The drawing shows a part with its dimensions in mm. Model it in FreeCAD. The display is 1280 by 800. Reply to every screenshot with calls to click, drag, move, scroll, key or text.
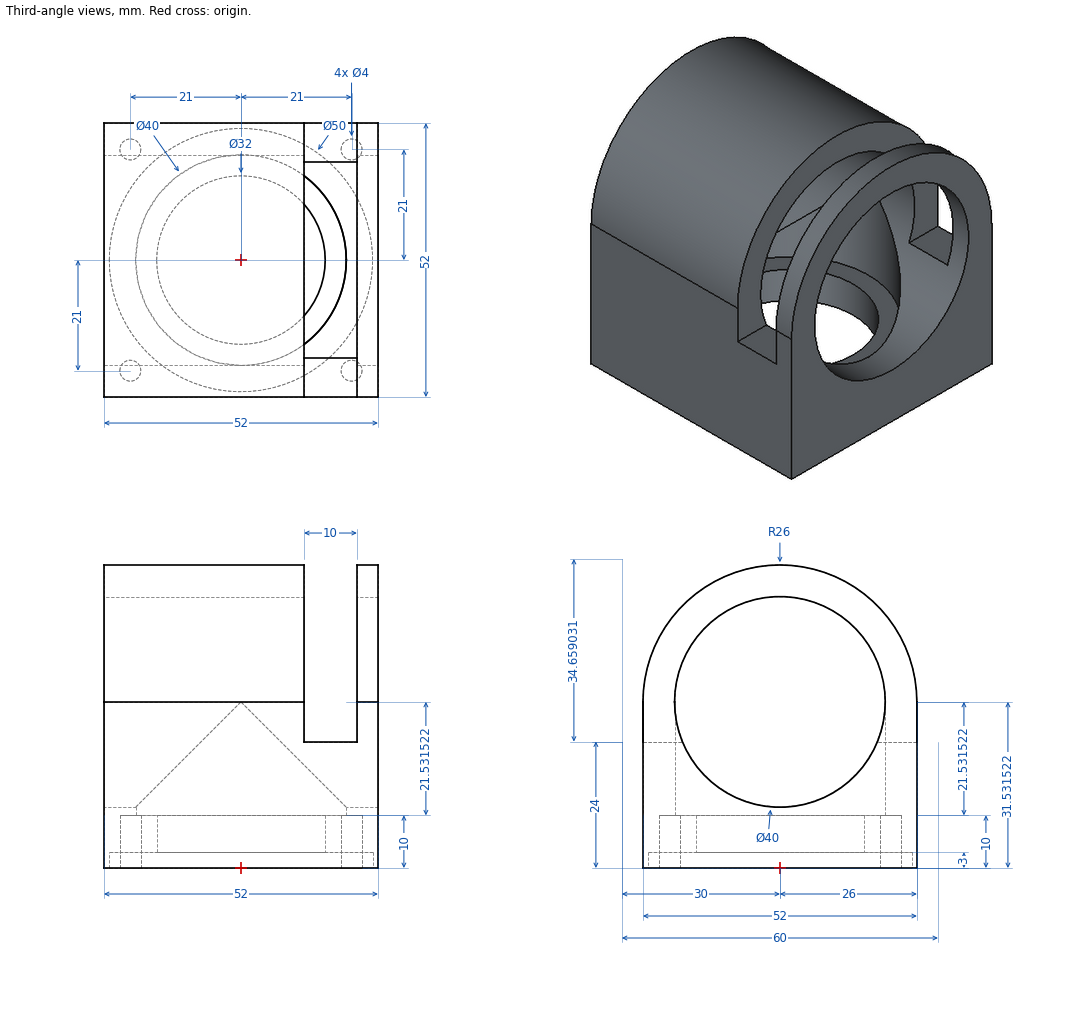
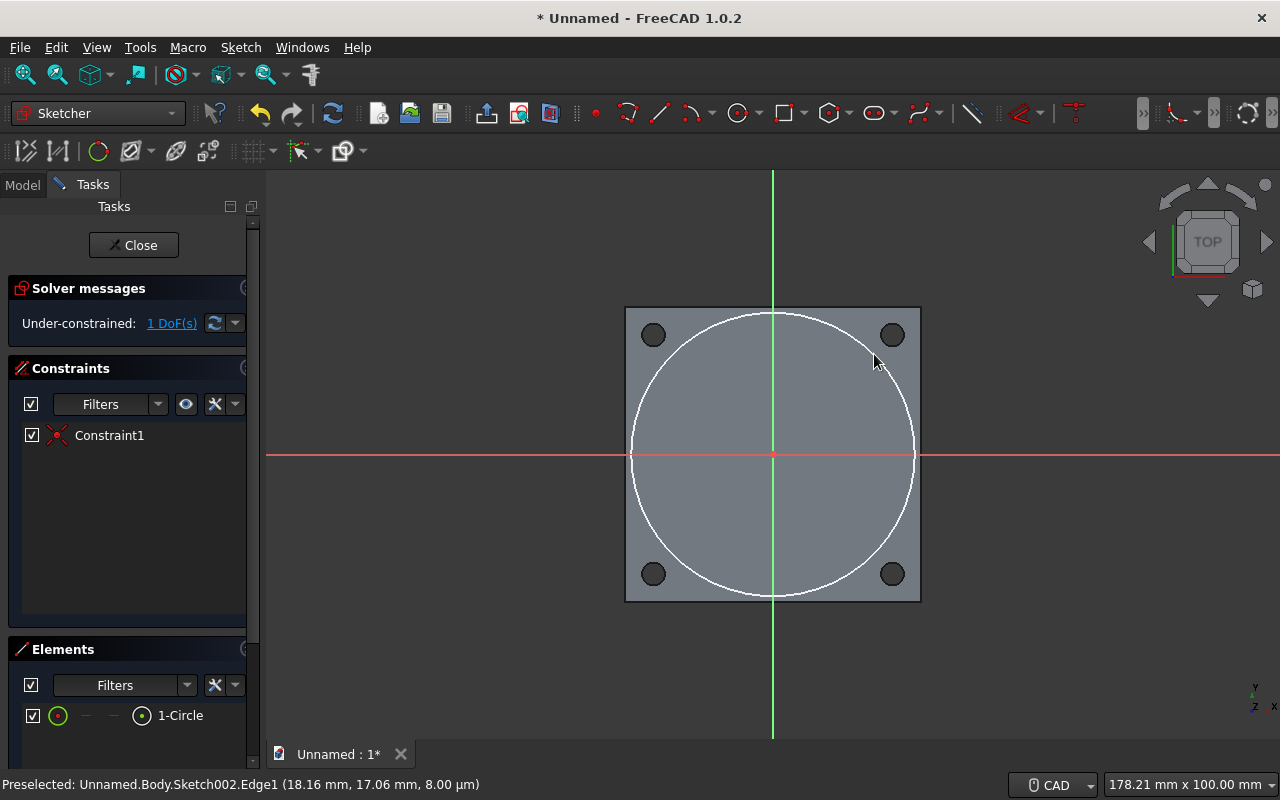
click(1020, 114)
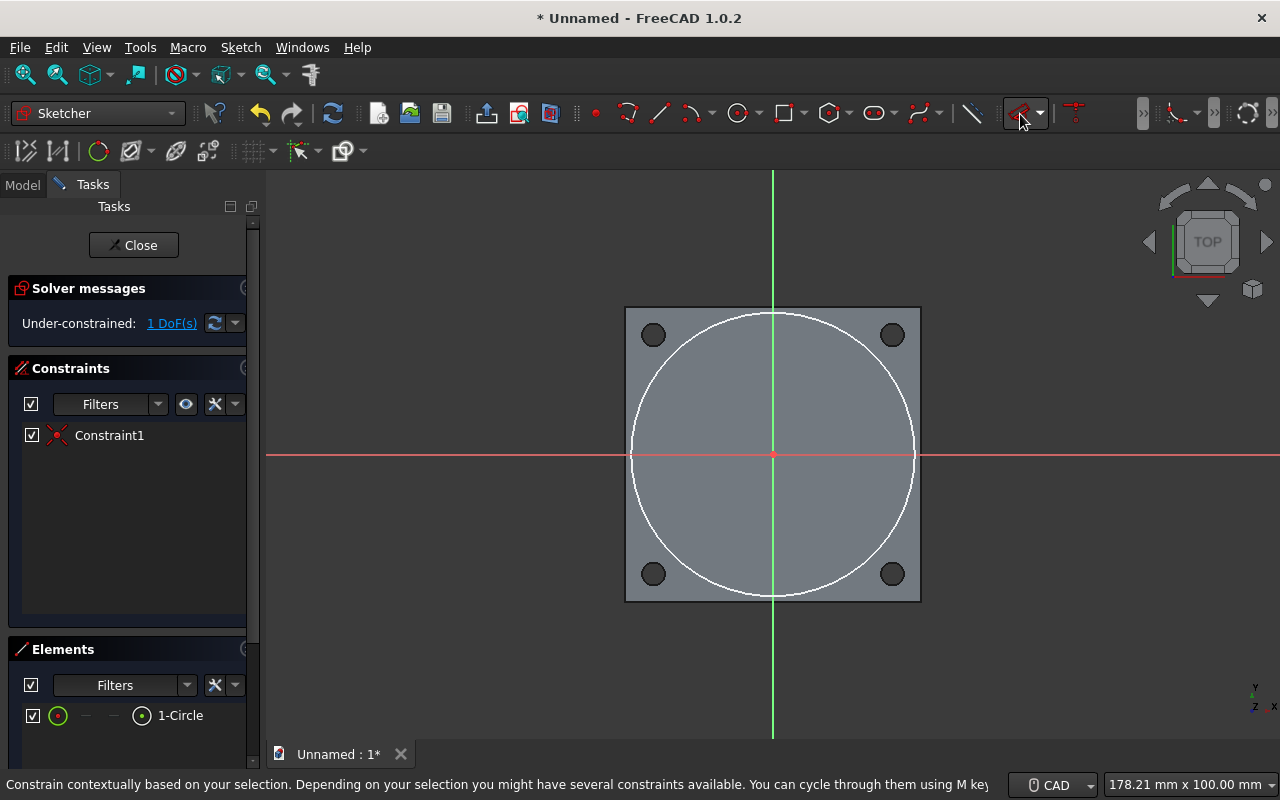
click(873, 354)
click(896, 331)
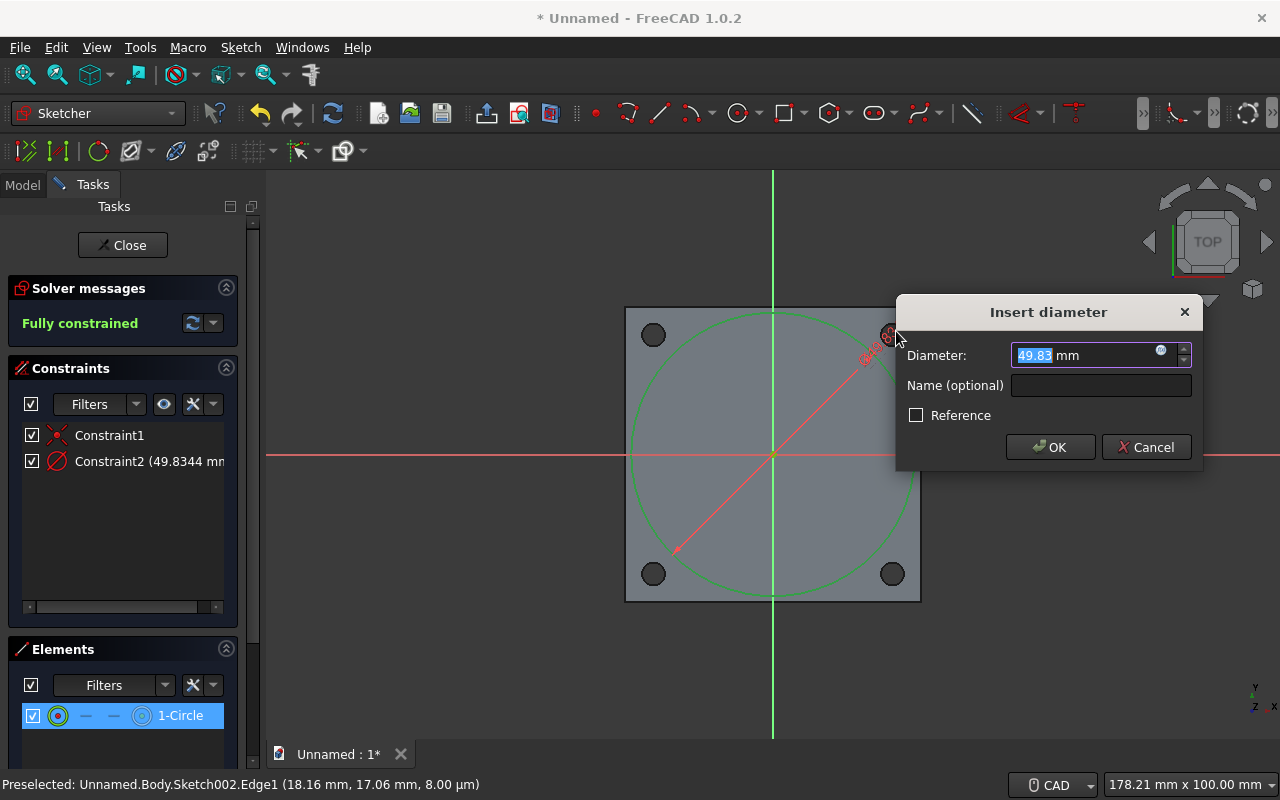
text(50)
key(Return)
key(Escape)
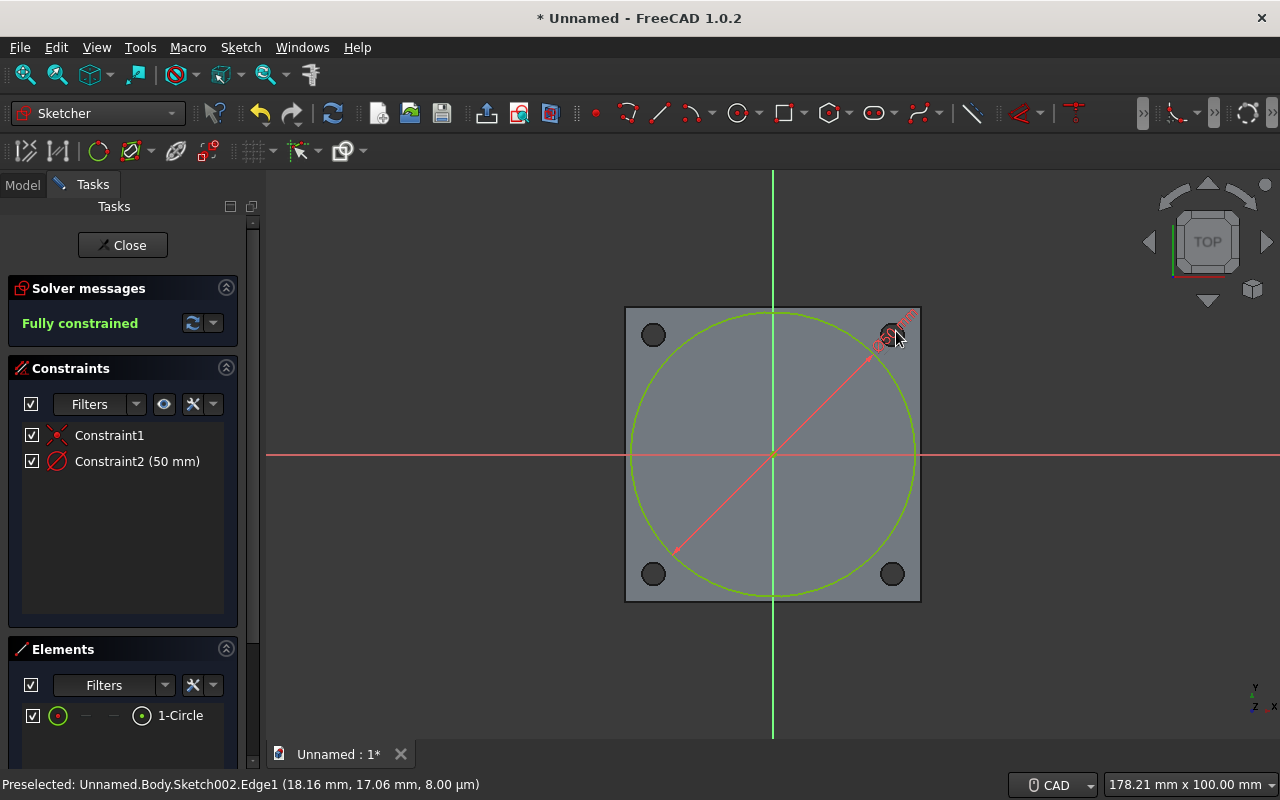
click(123, 245)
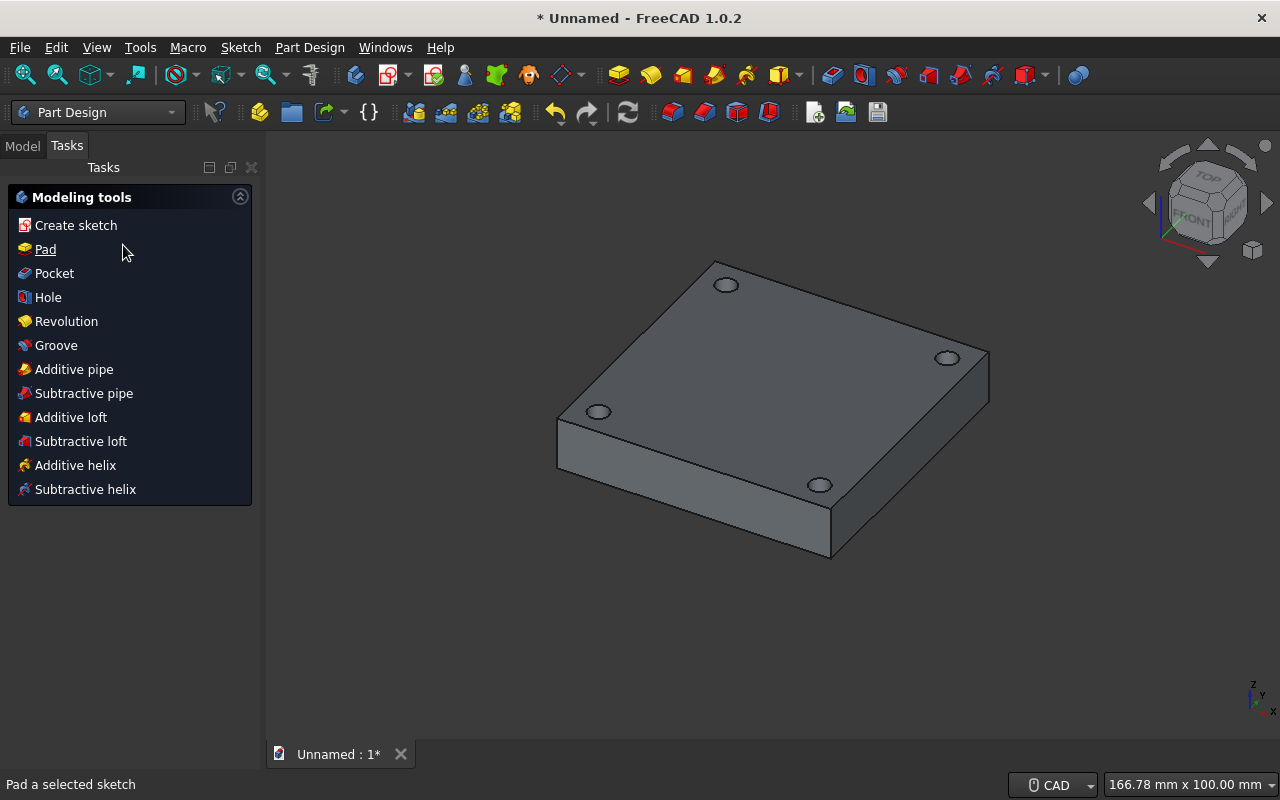
click(834, 76)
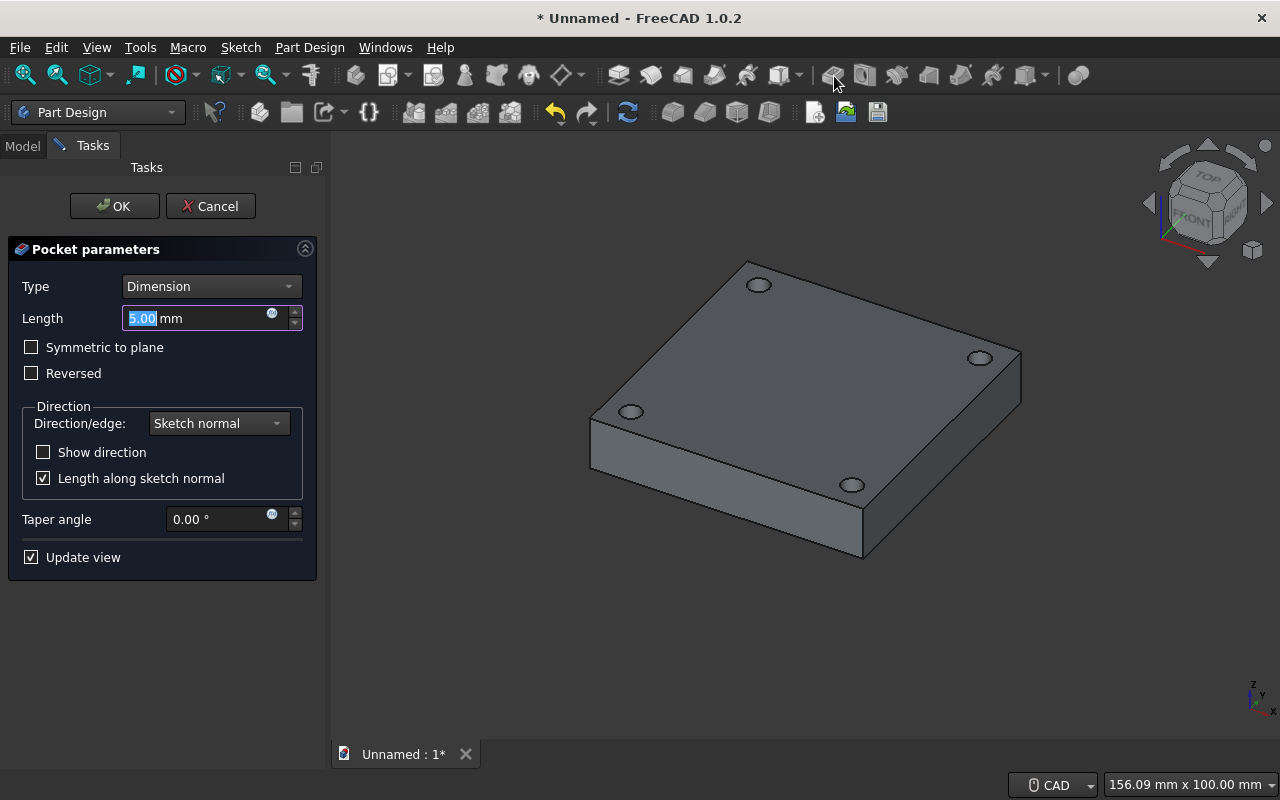
text(3)
key(Tab)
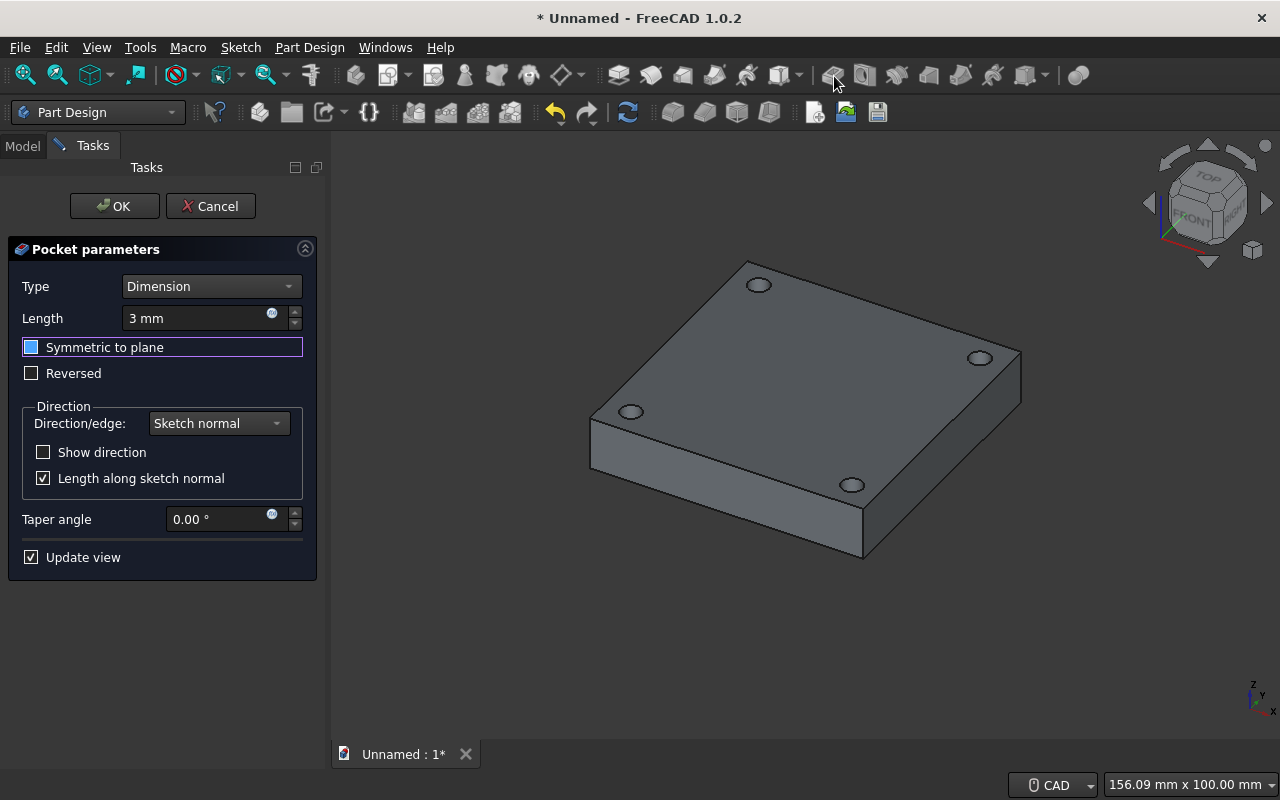
click(30, 373)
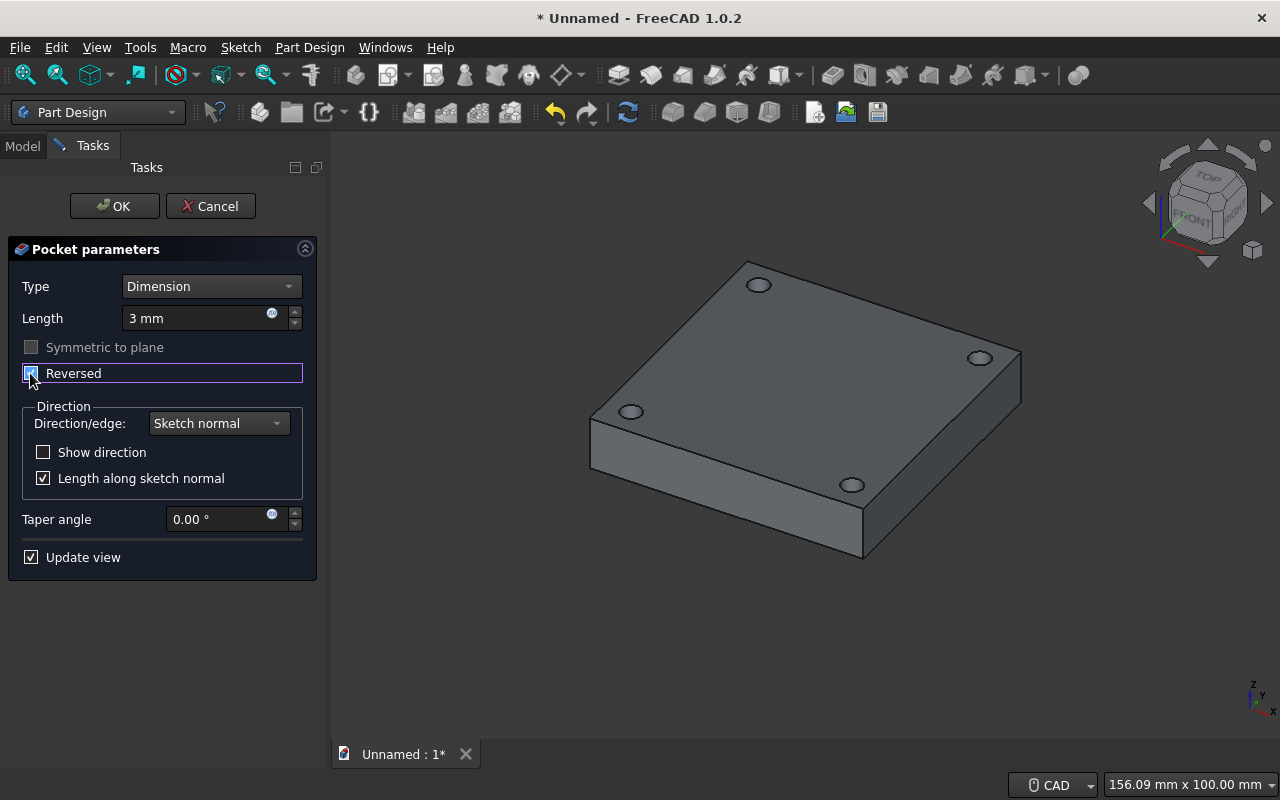
click(115, 206)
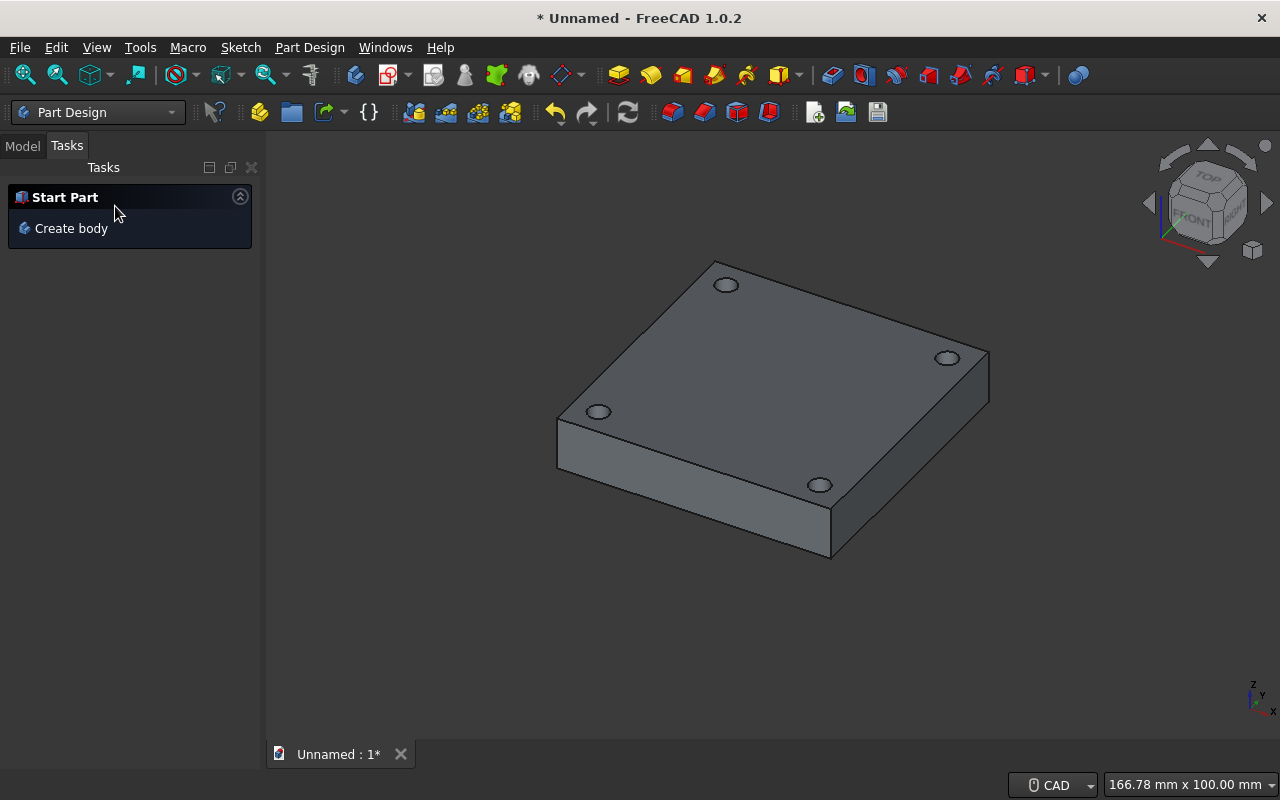
key(5)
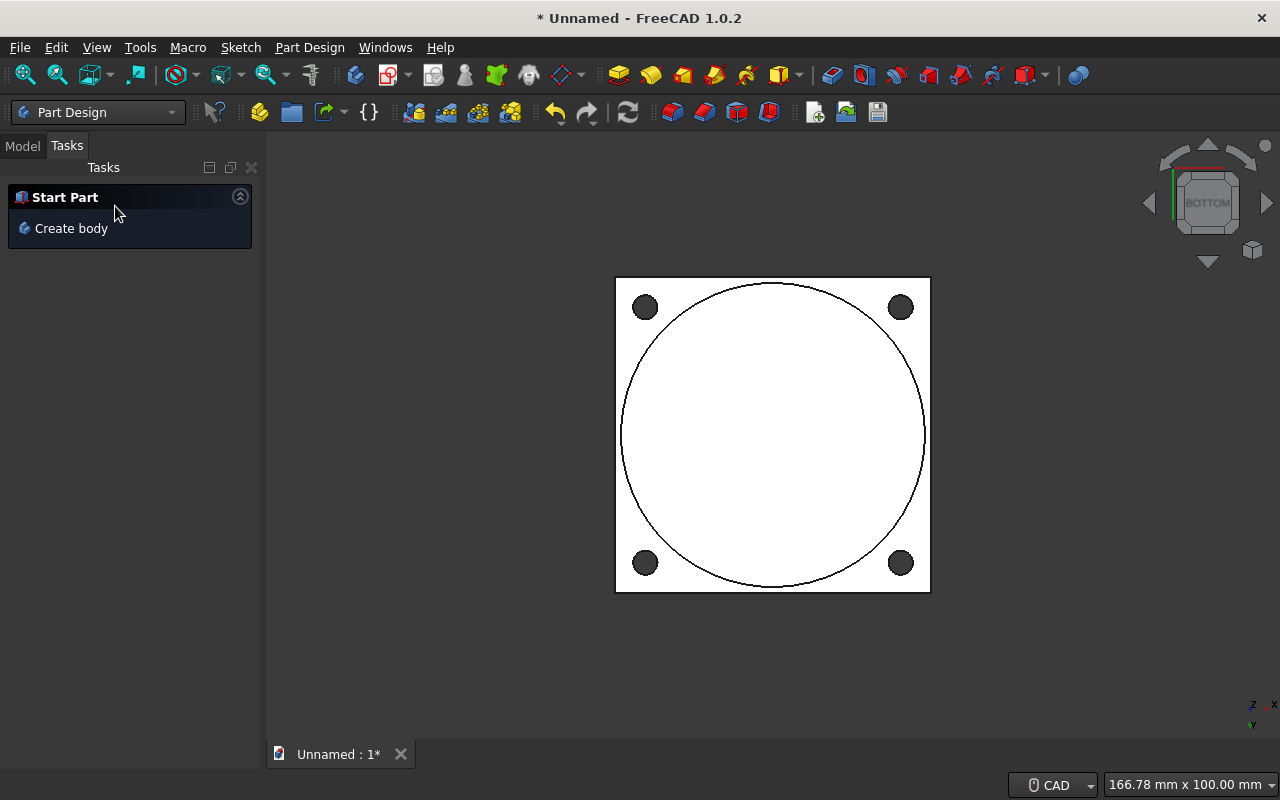
click(773, 434)